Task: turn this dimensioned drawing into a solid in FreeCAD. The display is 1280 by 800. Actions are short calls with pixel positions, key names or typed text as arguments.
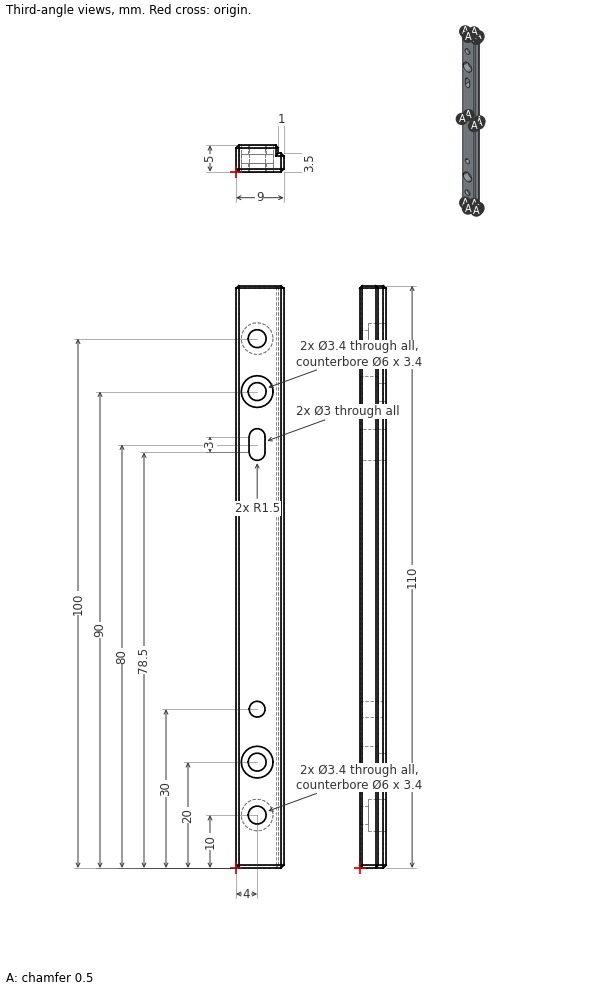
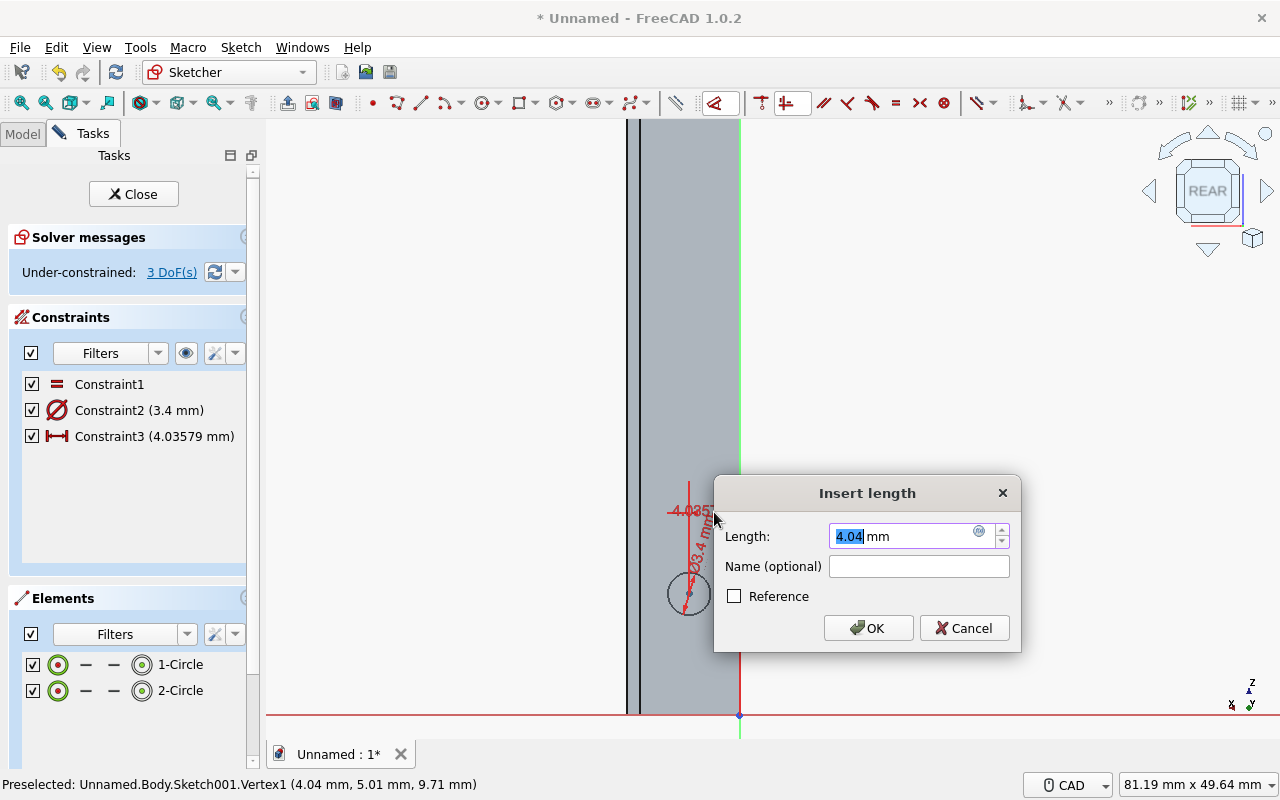
text(4)
key(Return)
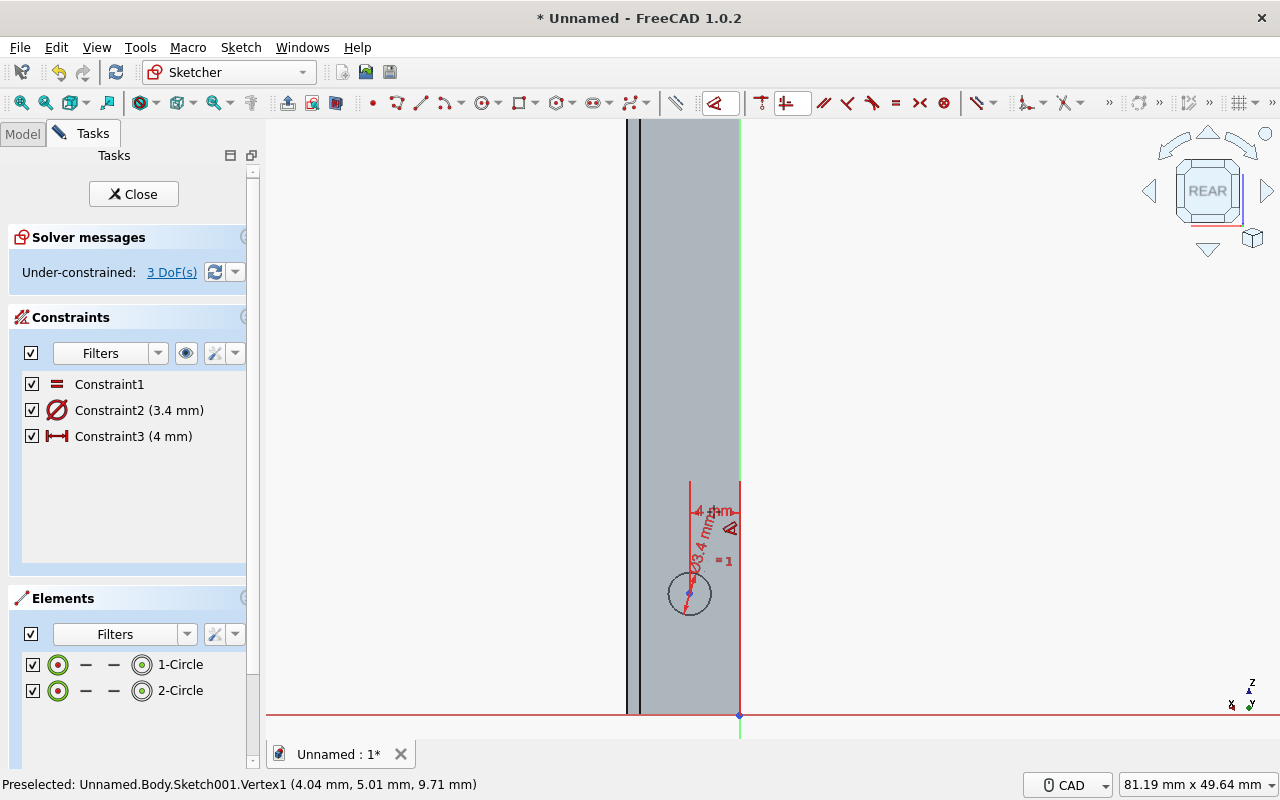
scroll(705, 579, down, 6)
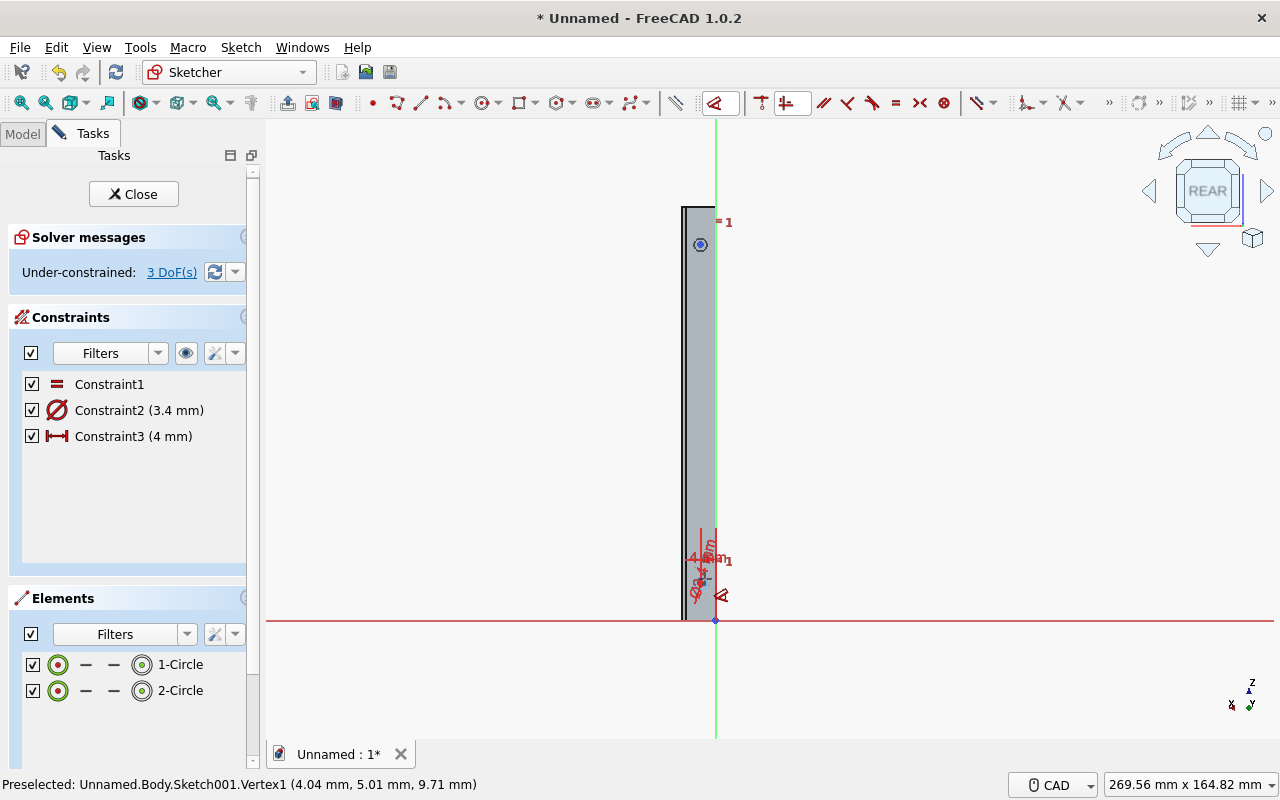
scroll(701, 245, up, 5)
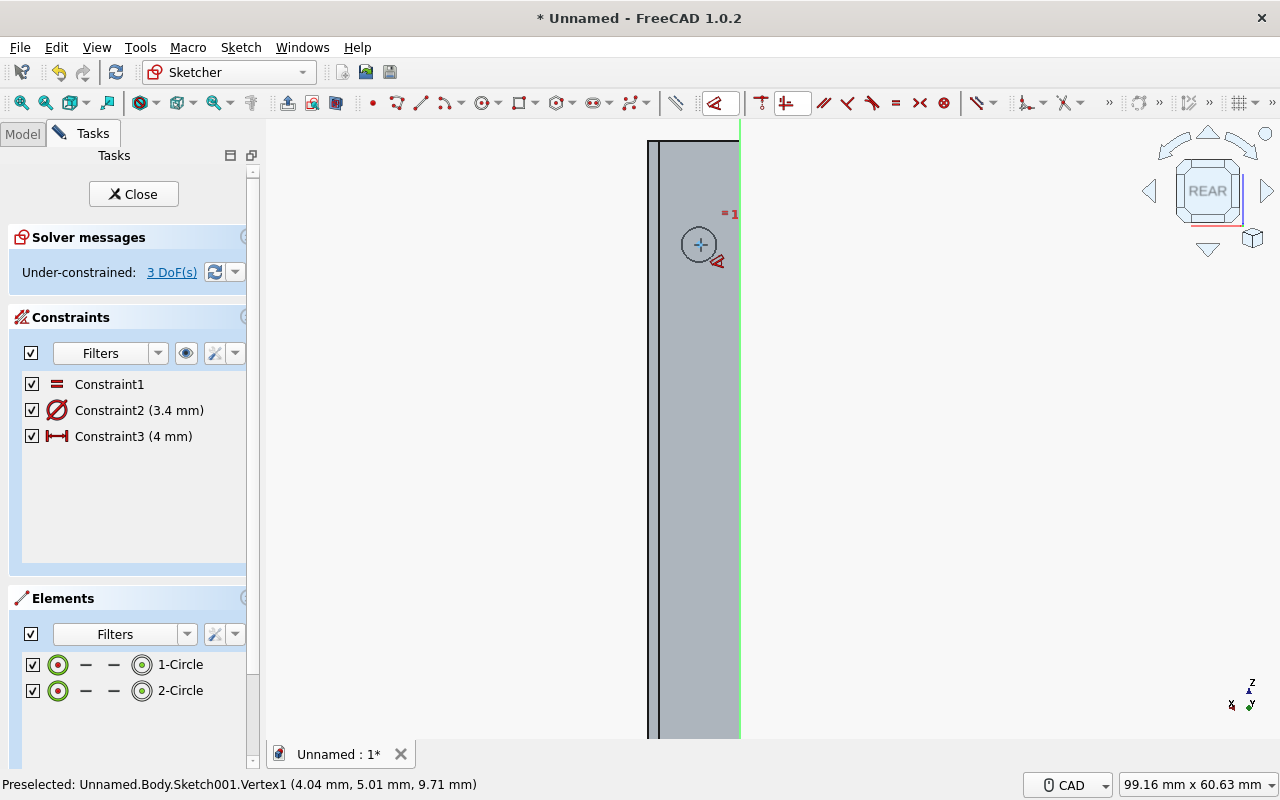
click(699, 245)
click(720, 211)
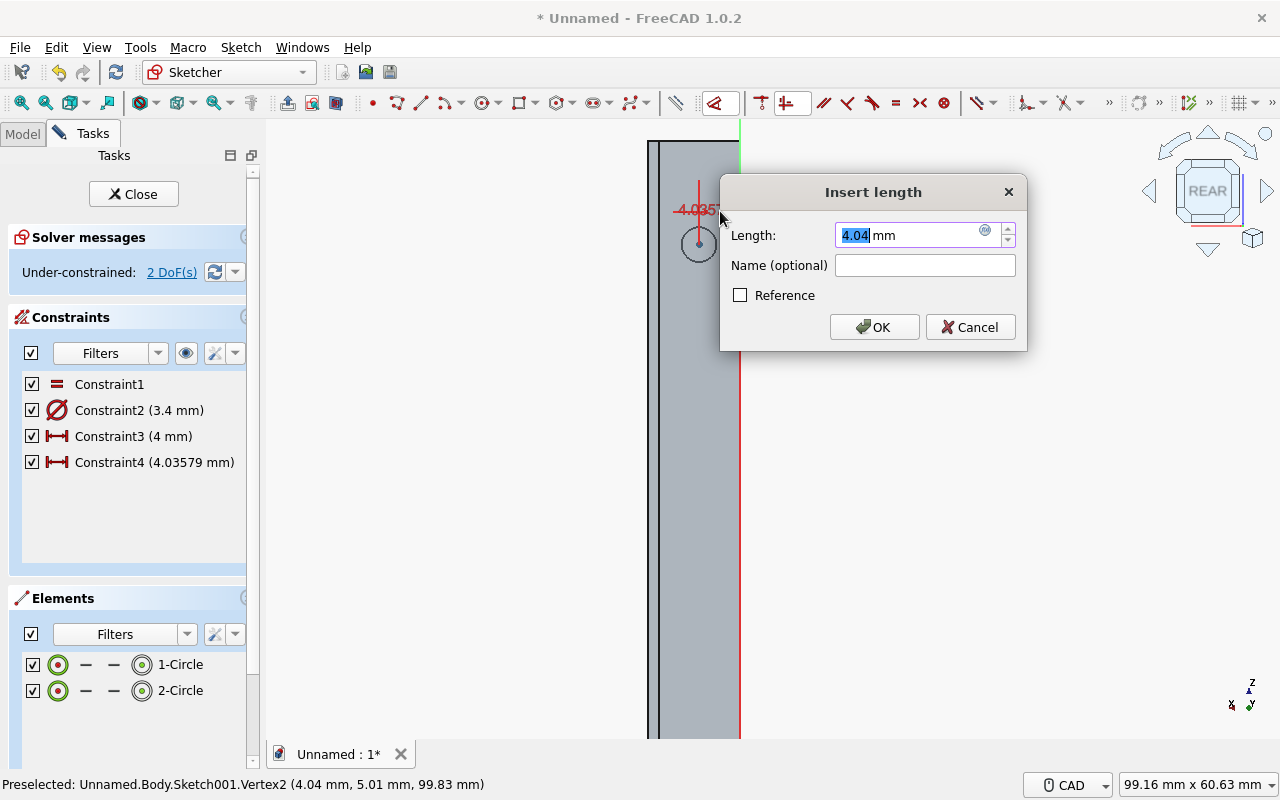
text(4)
key(Return)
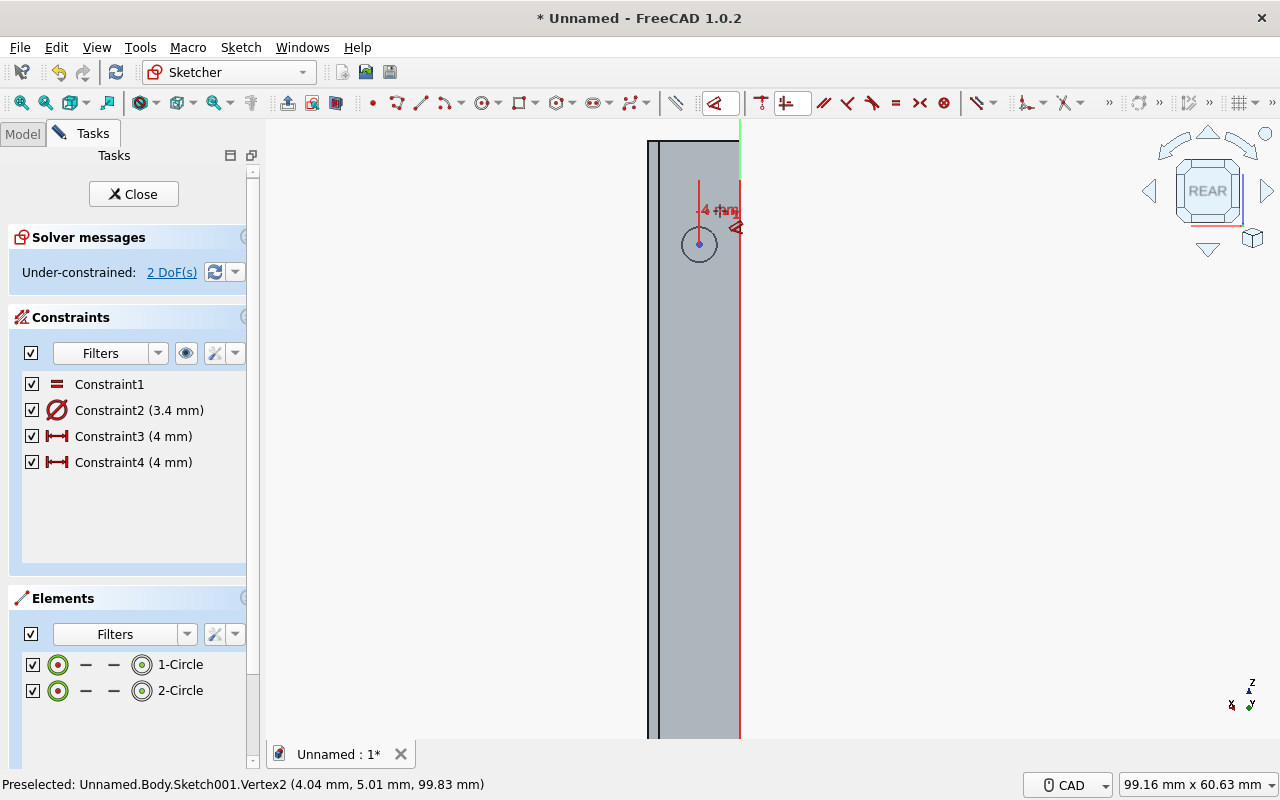
scroll(701, 245, down, 5)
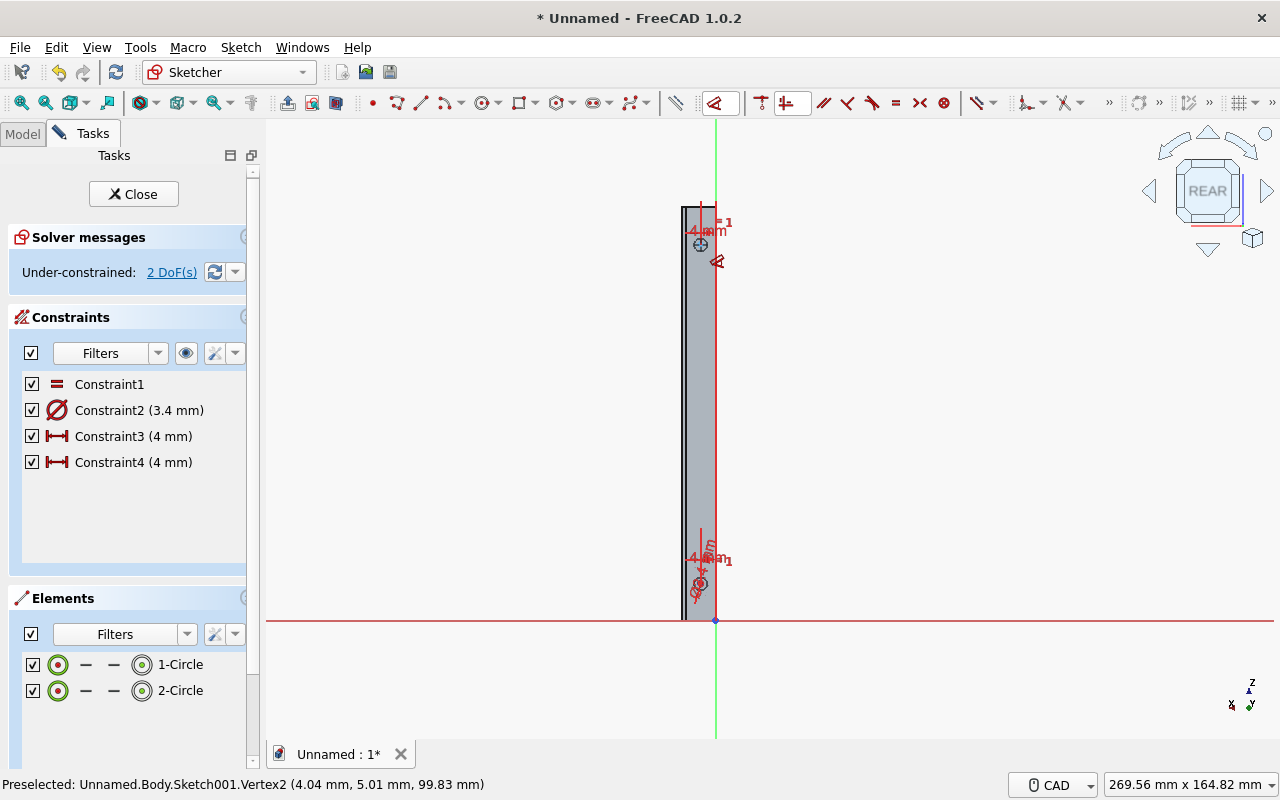
click(701, 584)
click(750, 602)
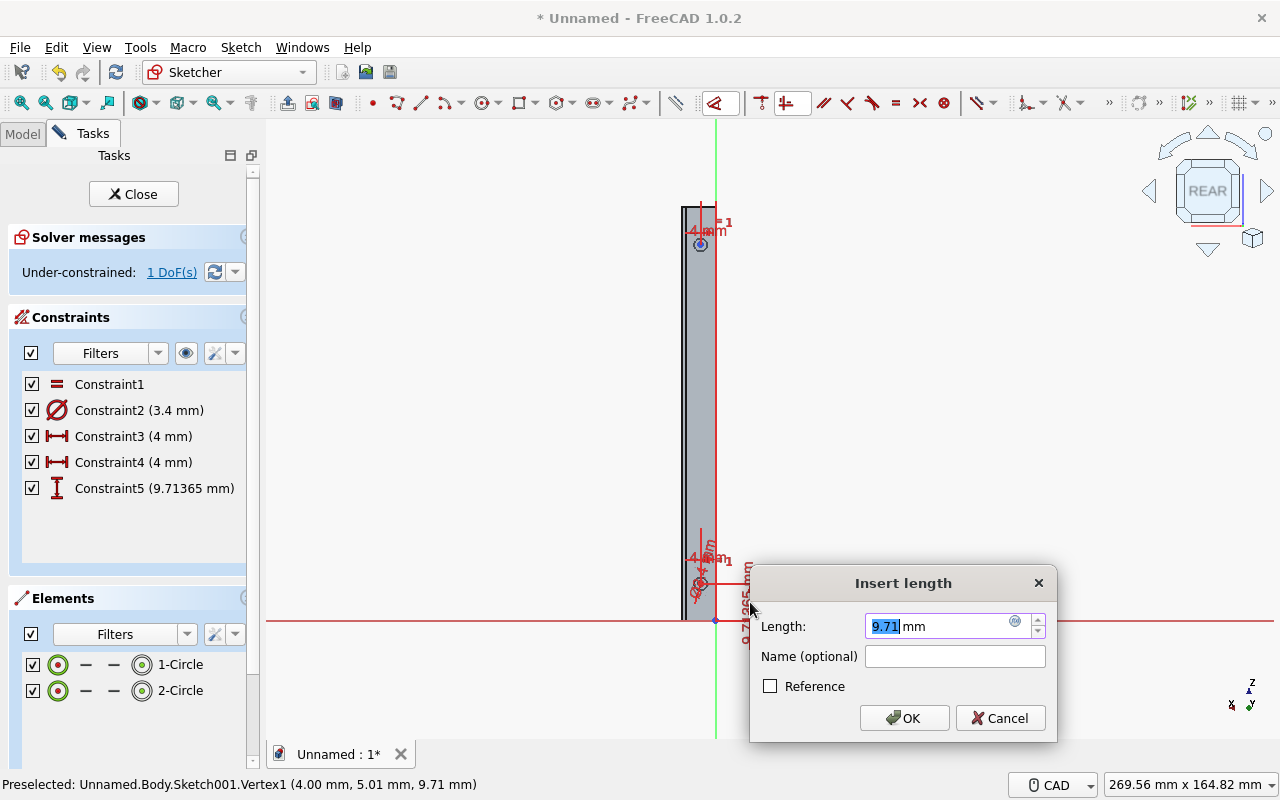
text(10)
key(Return)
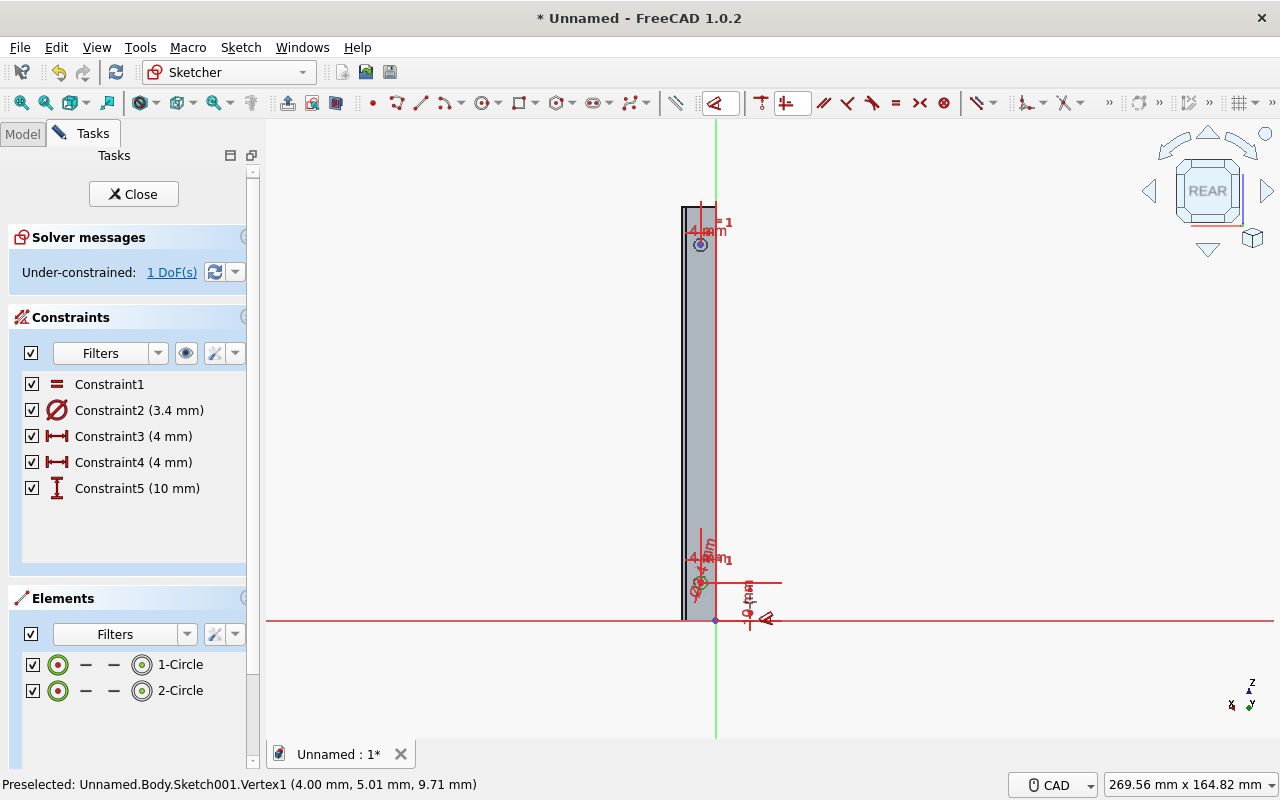
click(701, 245)
click(750, 433)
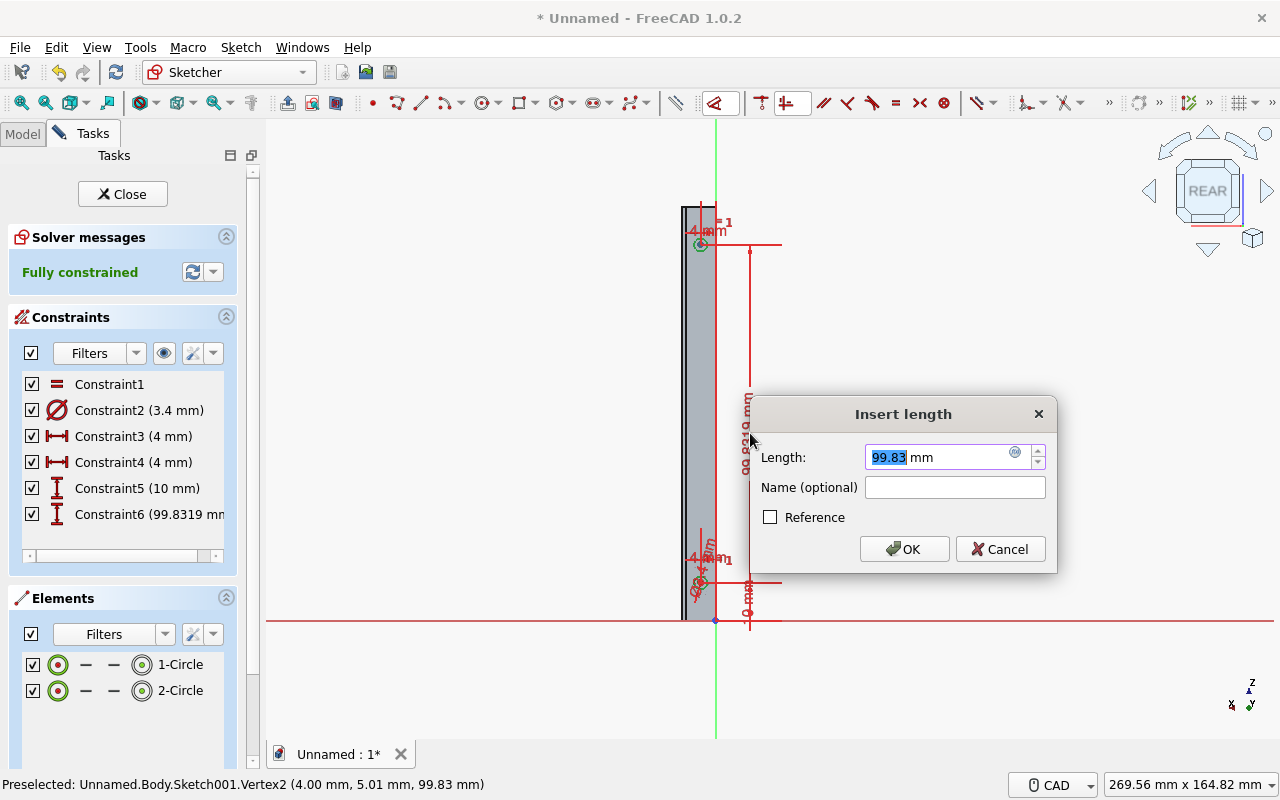
text(100)
key(Return)
key(Escape)